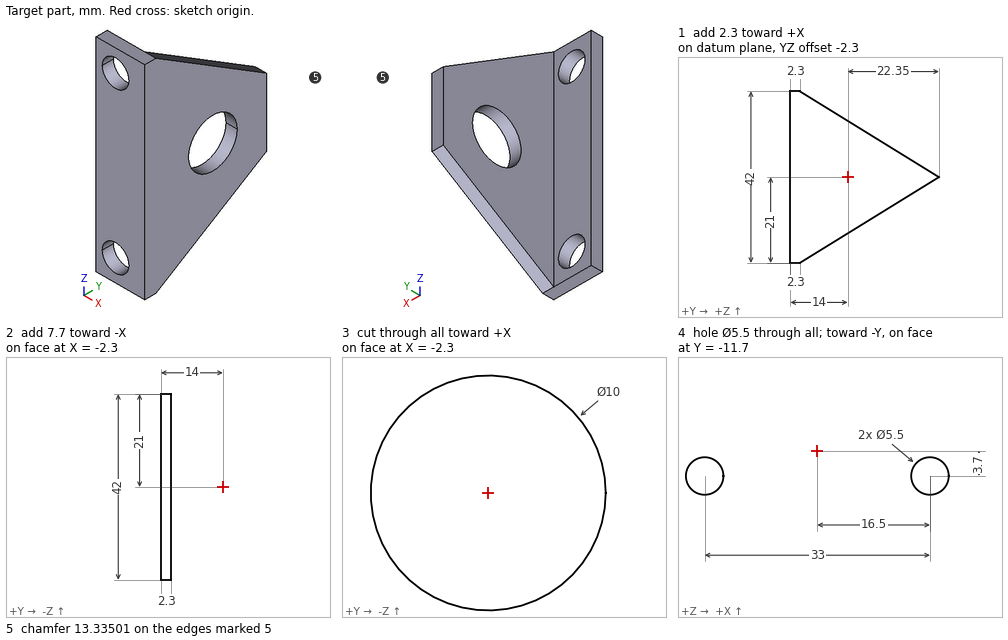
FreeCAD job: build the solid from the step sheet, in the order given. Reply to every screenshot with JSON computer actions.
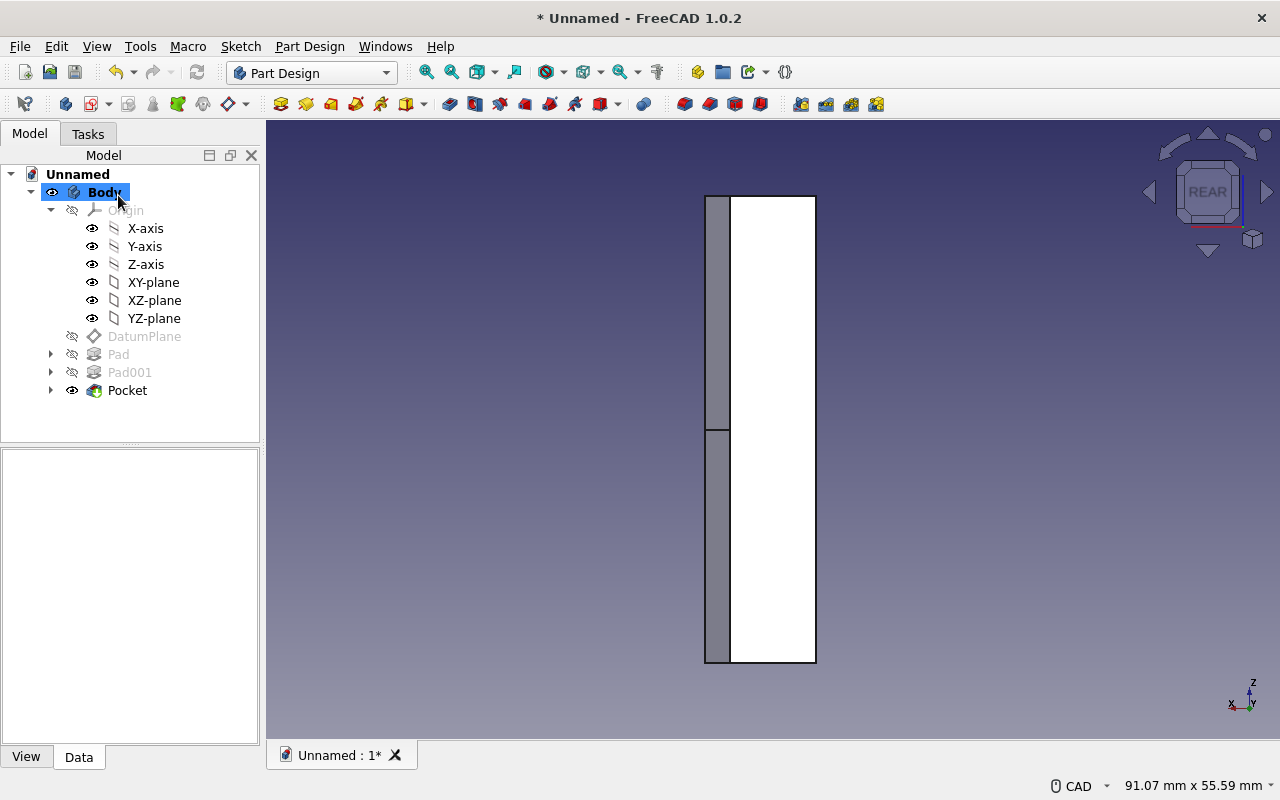
{"action": "left_click", "coordinate": [773, 295]}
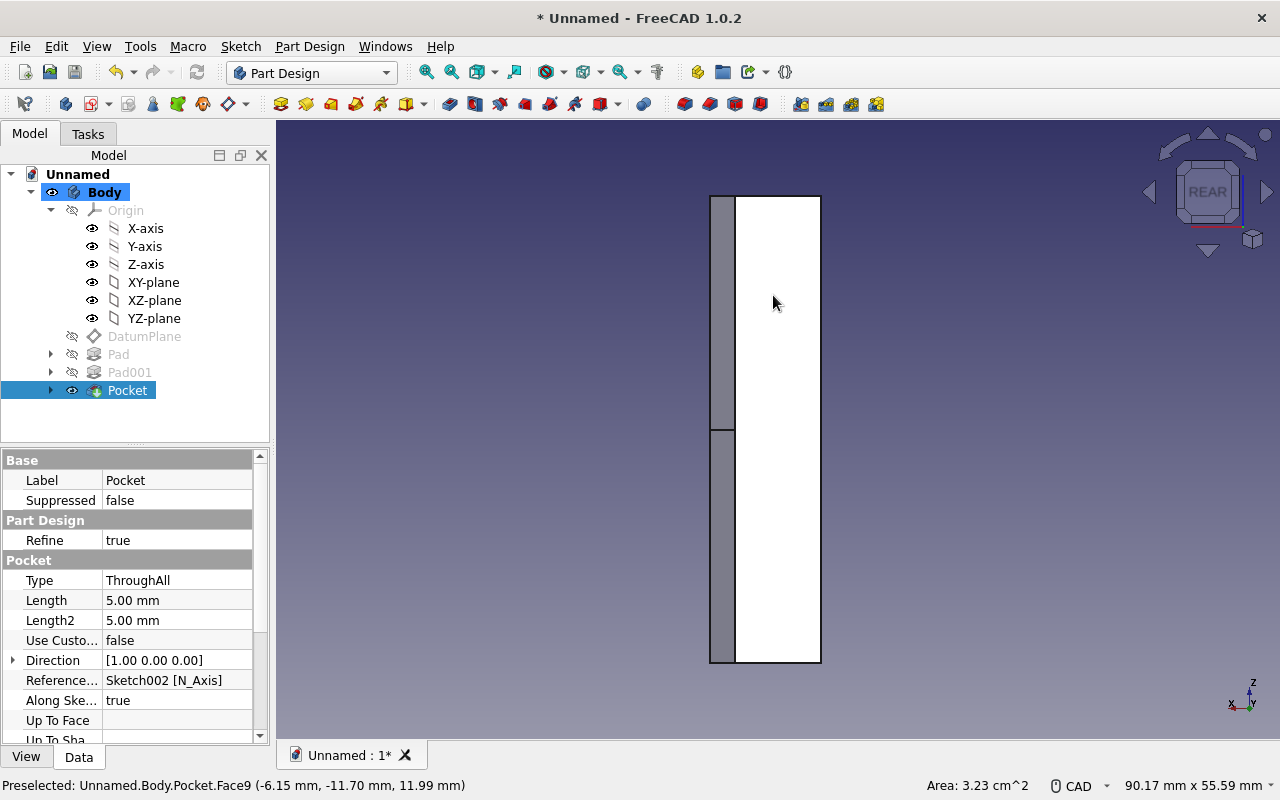
{"action": "left_click", "coordinate": [90, 104]}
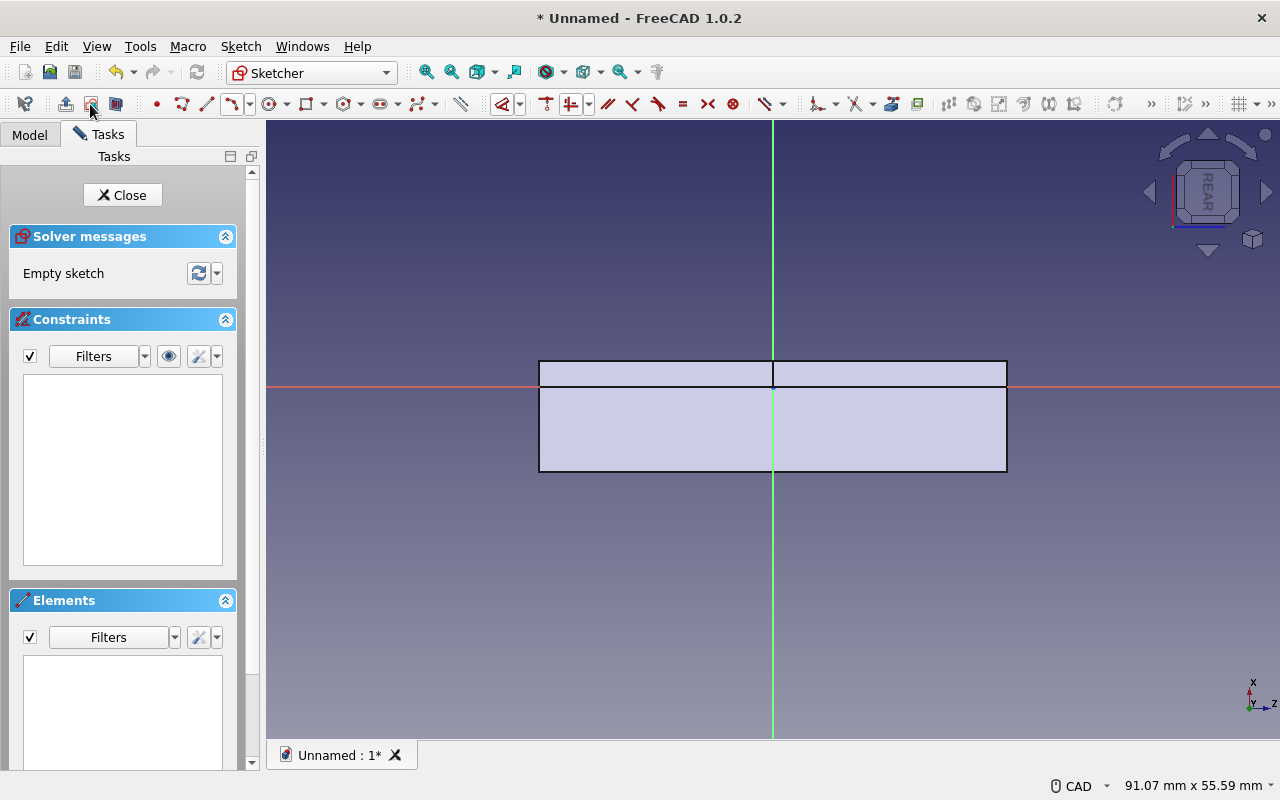
{"action": "key", "text": "q s"}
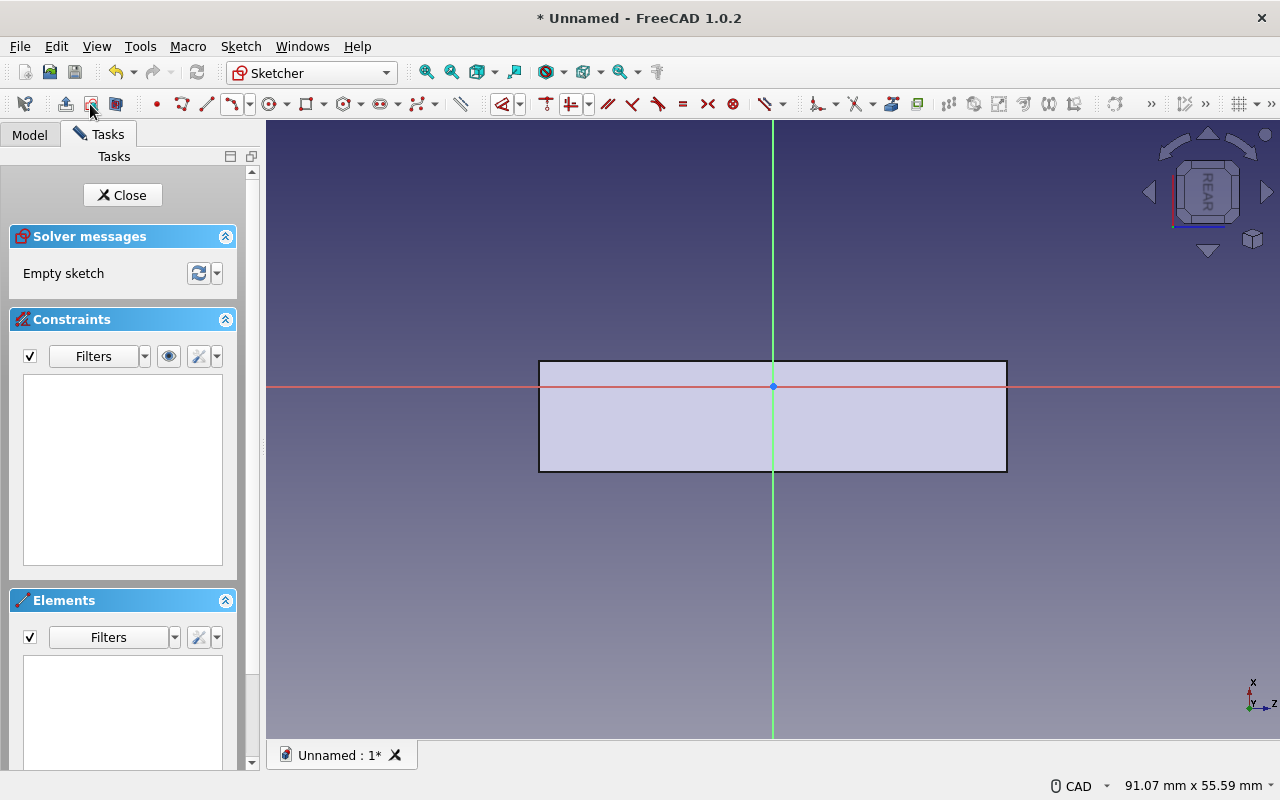
{"action": "scroll", "coordinate": [912, 408], "scroll_direction": "up", "scroll_amount": 2}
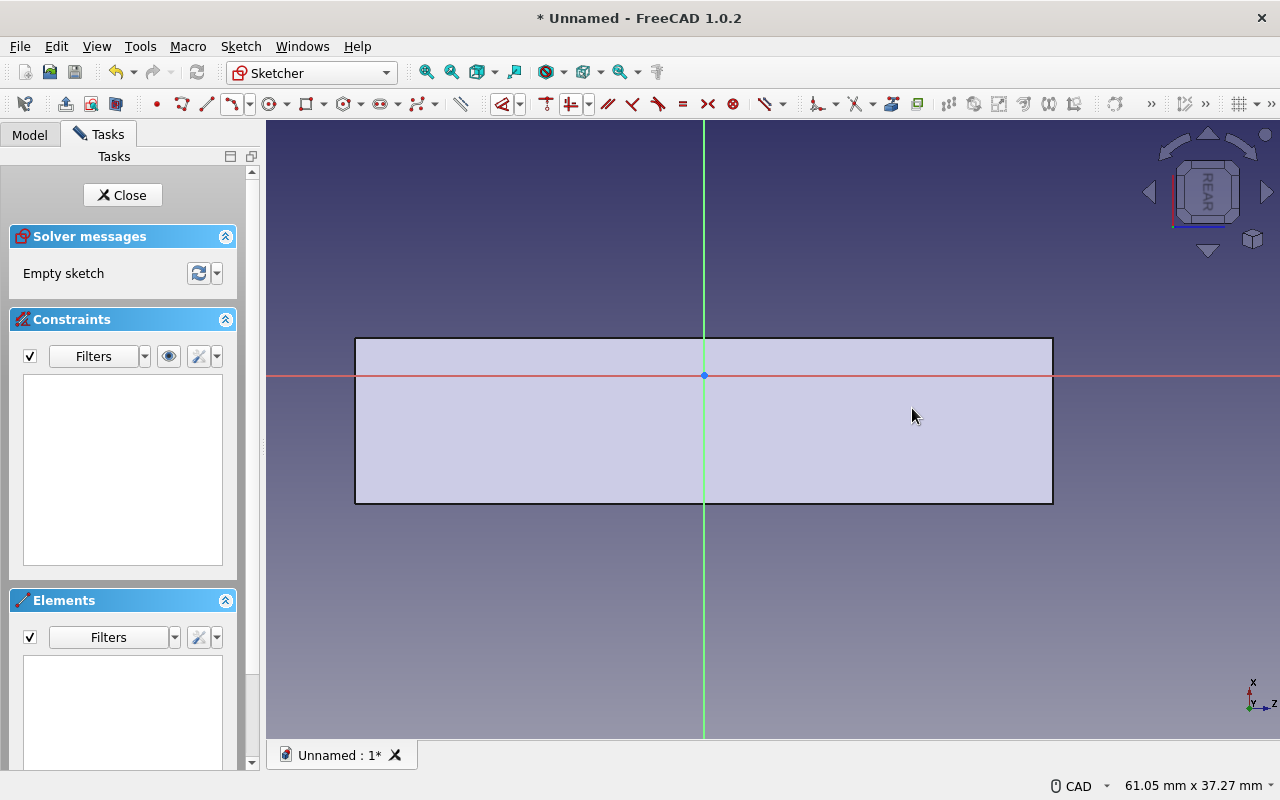
{"action": "key", "text": "g c"}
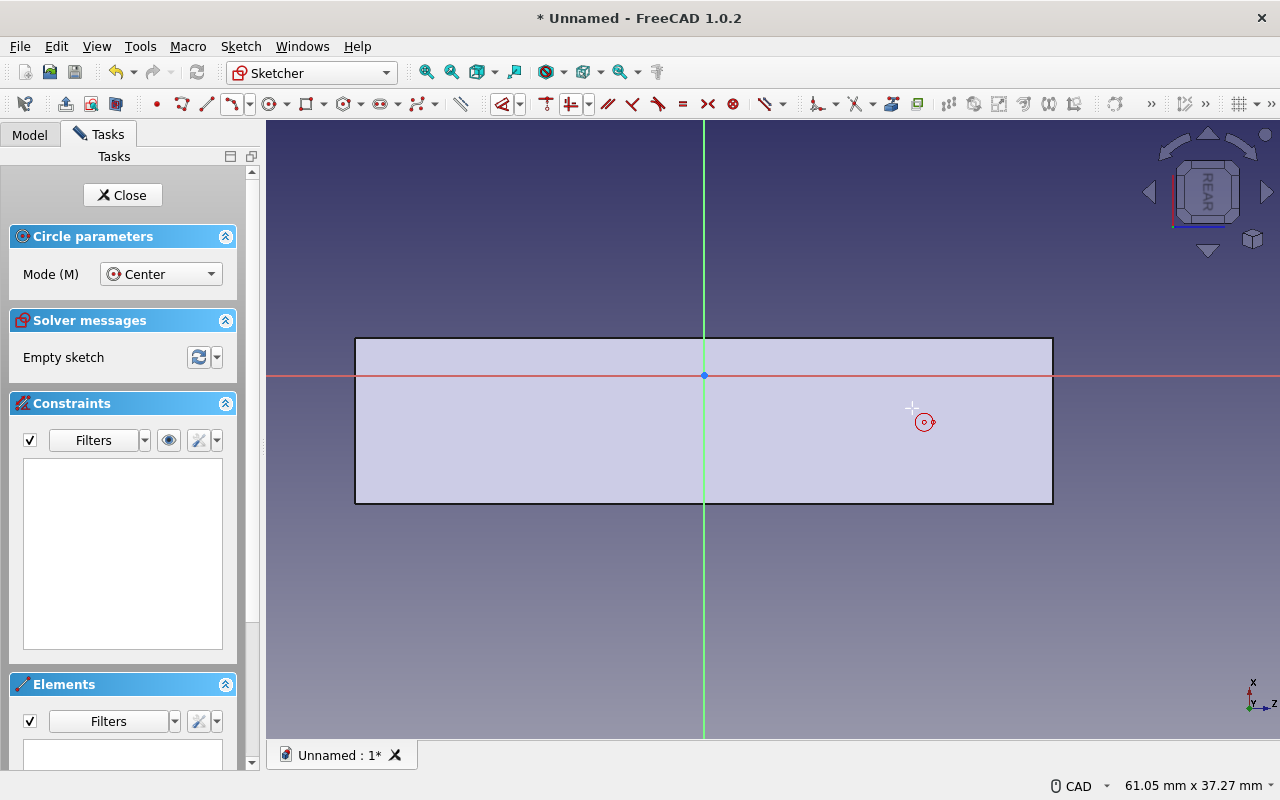
{"action": "left_click", "coordinate": [978, 437]}
{"action": "left_click", "coordinate": [1011, 405]}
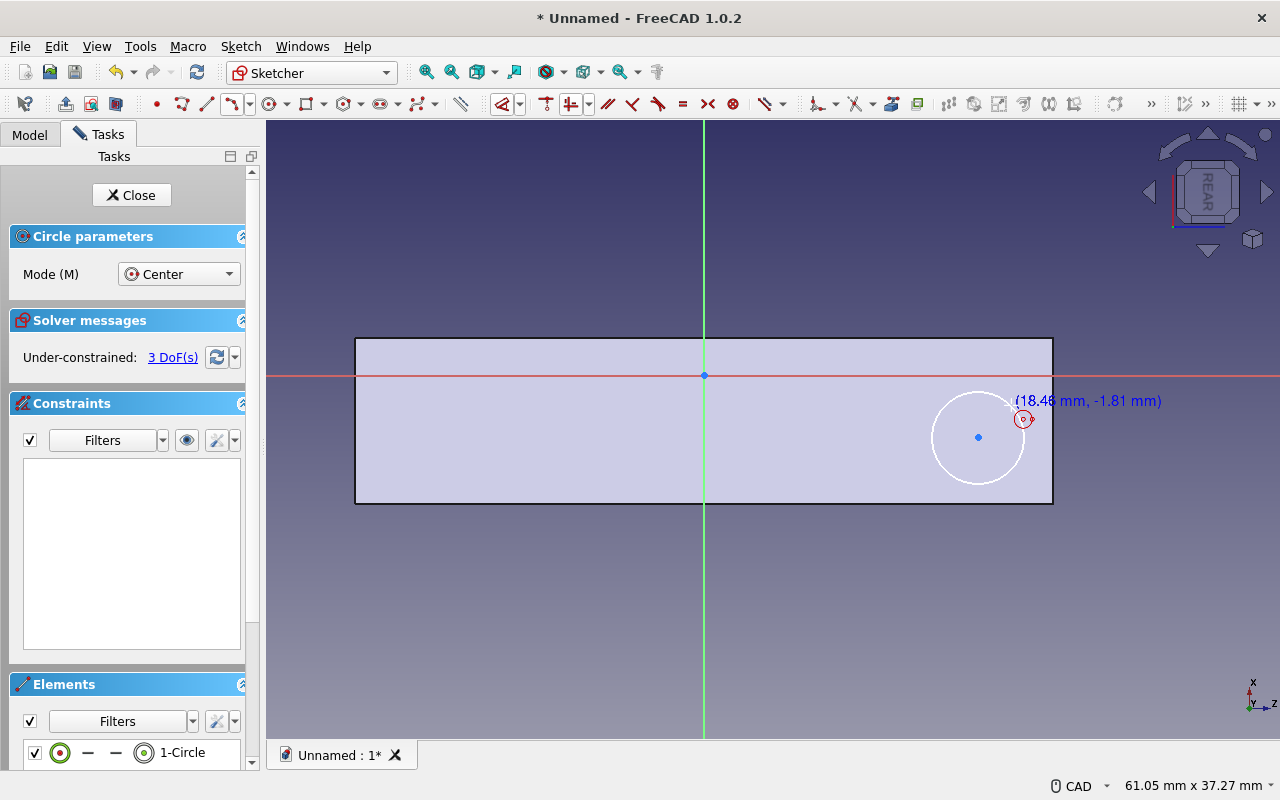
{"action": "left_click", "coordinate": [430, 437]}
{"action": "left_click", "coordinate": [463, 405]}
{"action": "key", "text": "Escape"}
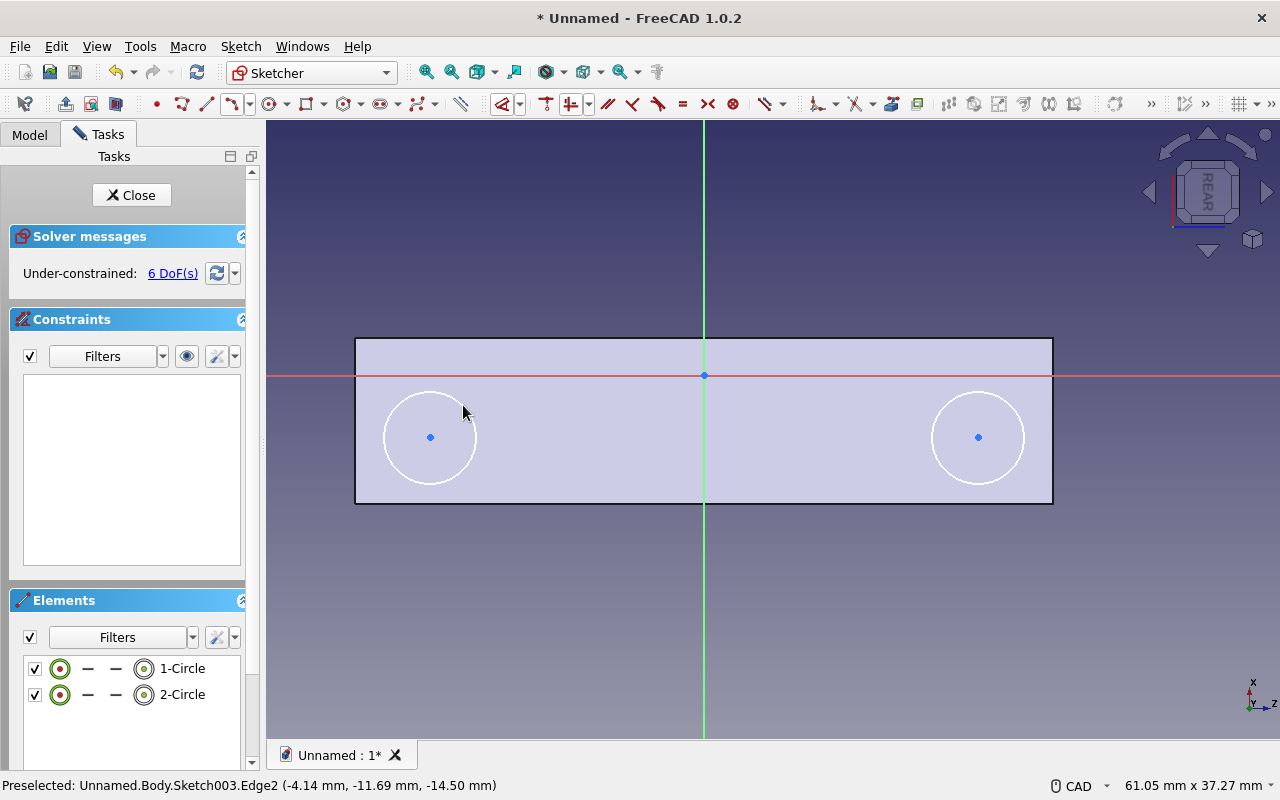
{"action": "left_click", "coordinate": [1010, 405]}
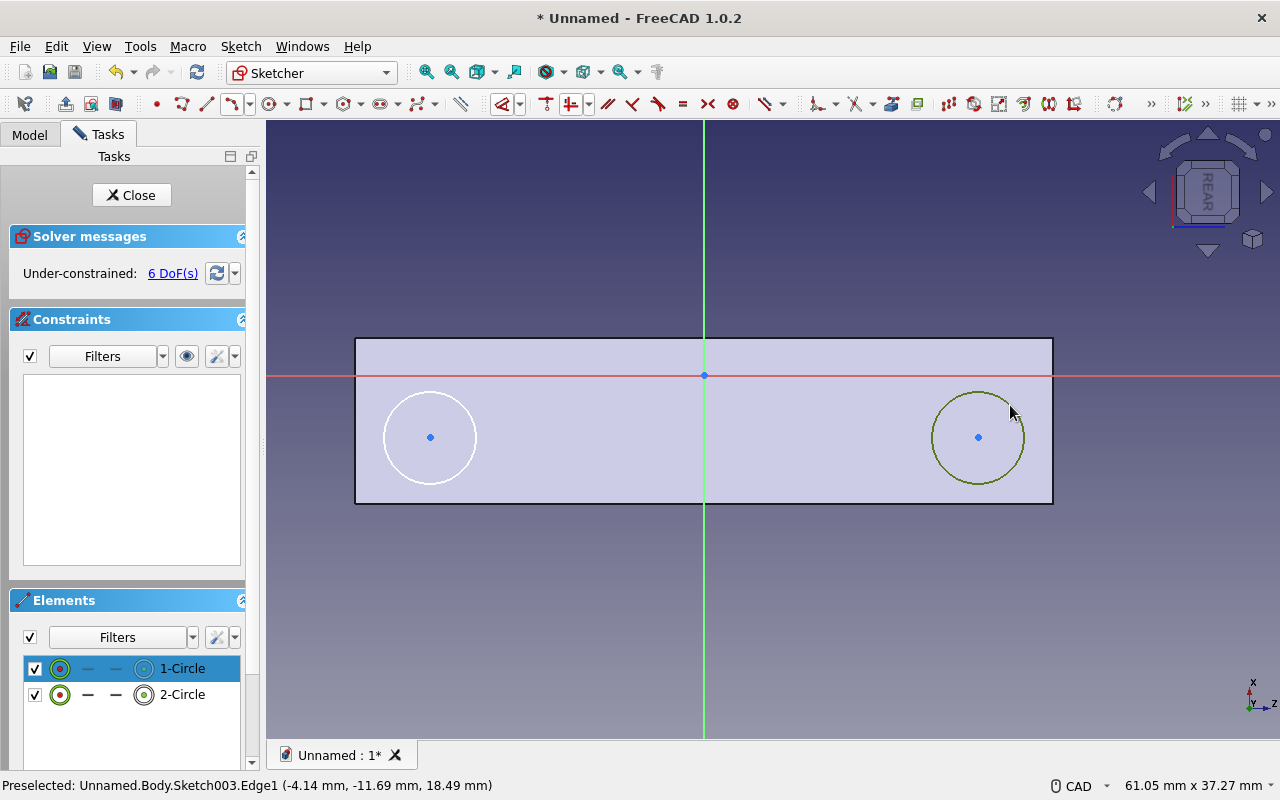
{"action": "left_click", "coordinate": [462, 405]}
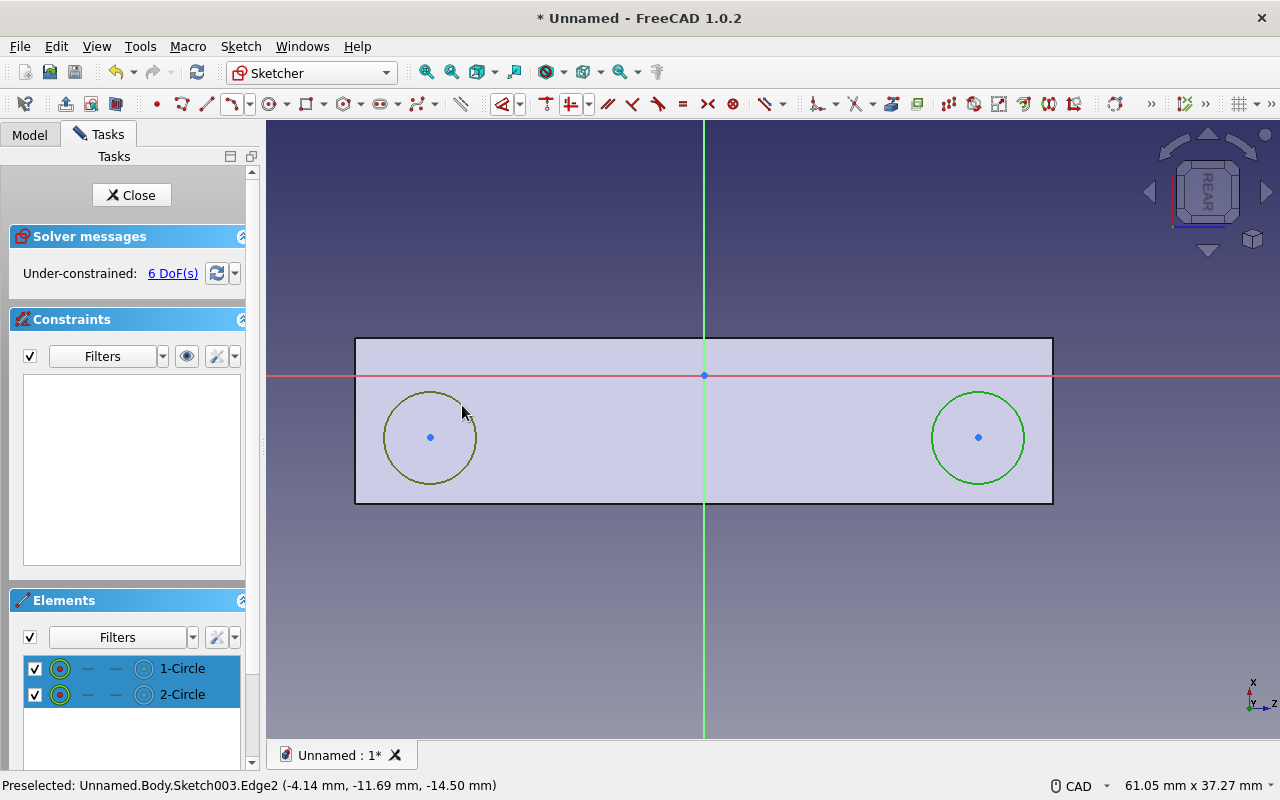
{"action": "key", "text": "e"}